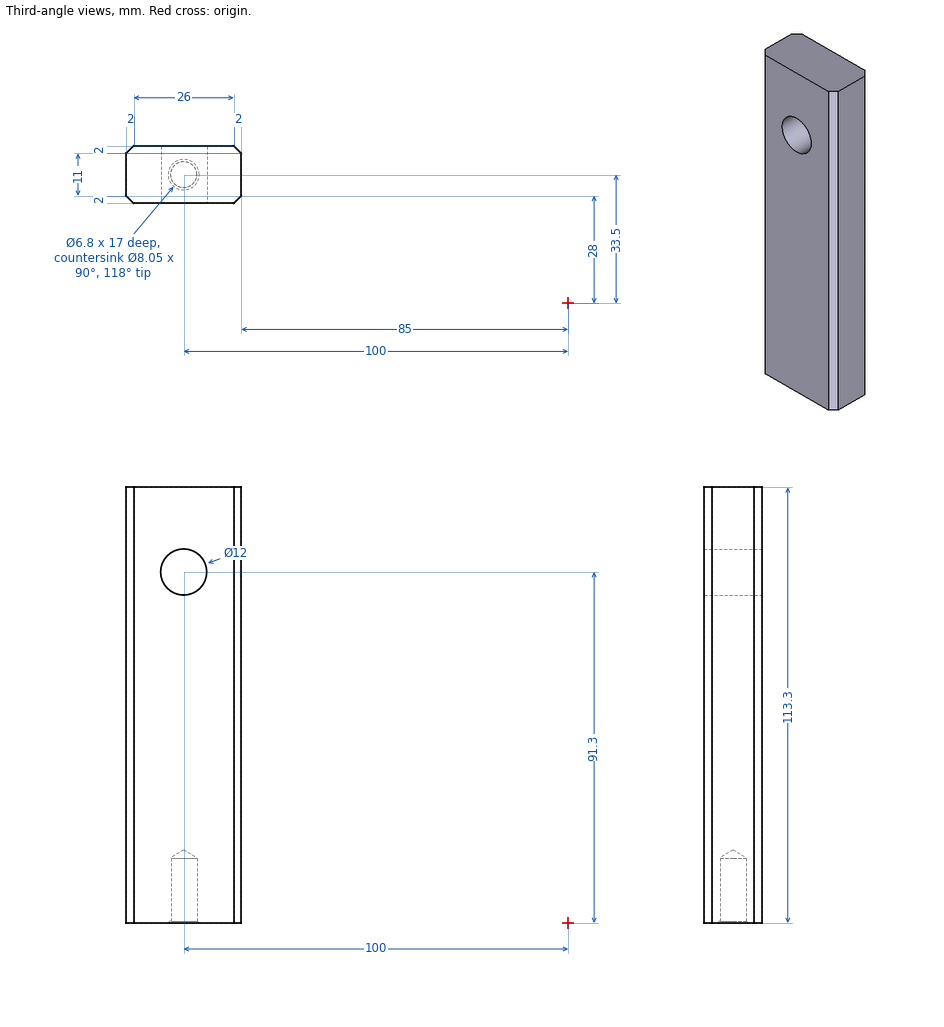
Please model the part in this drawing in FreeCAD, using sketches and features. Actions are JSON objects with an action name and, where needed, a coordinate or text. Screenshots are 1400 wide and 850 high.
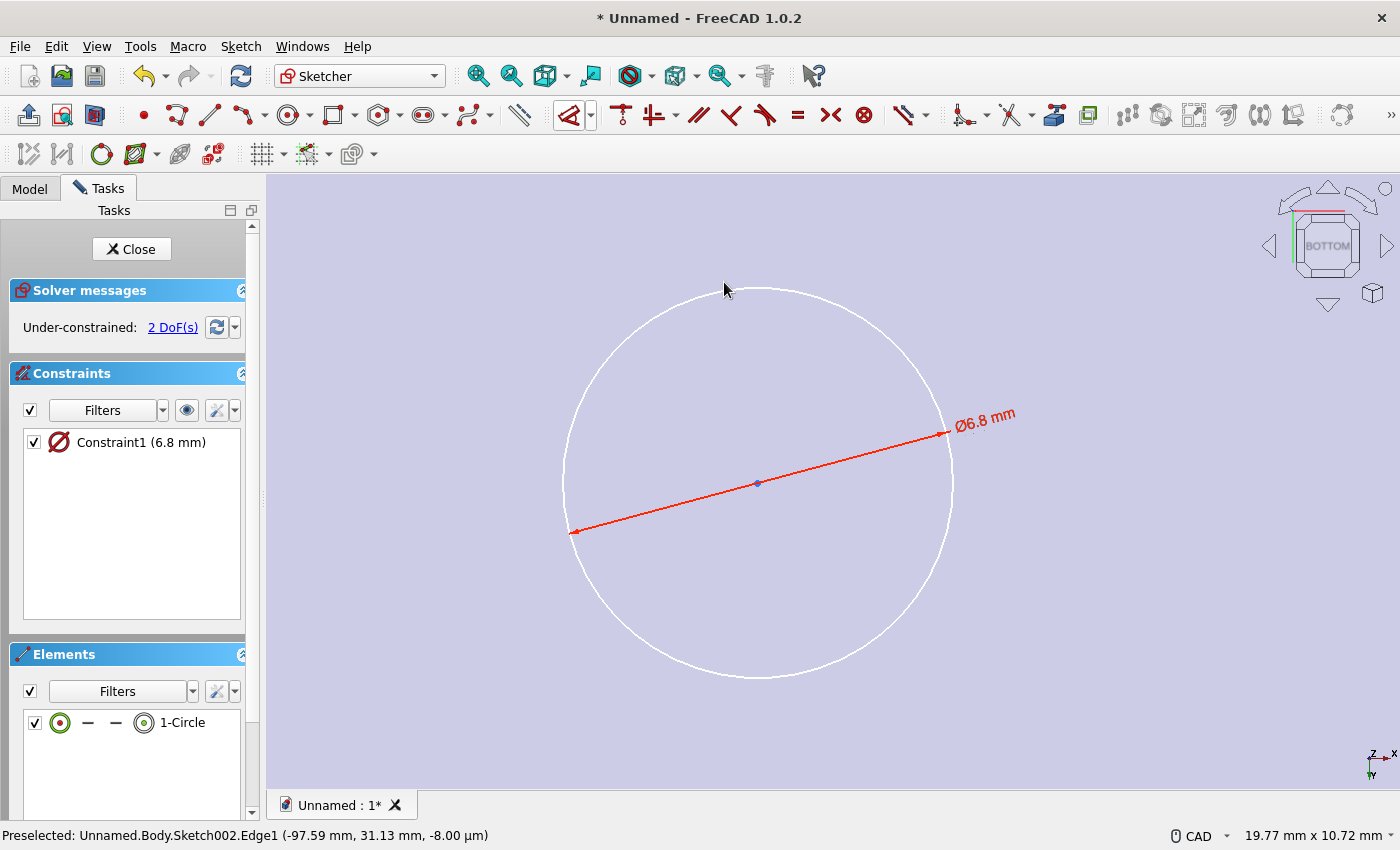
{"action": "left_click", "coordinate": [758, 483]}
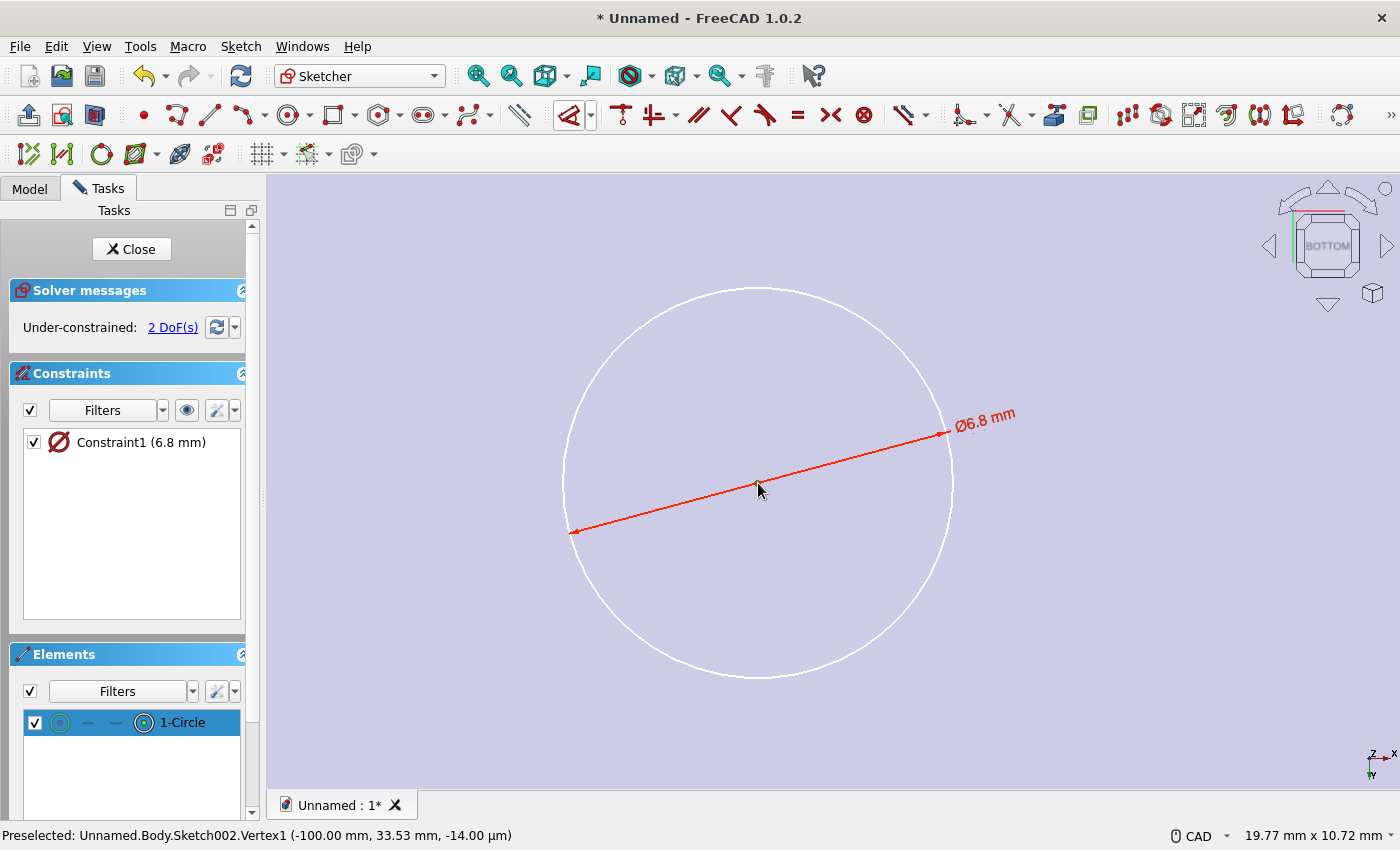
{"action": "left_click", "coordinate": [590, 116]}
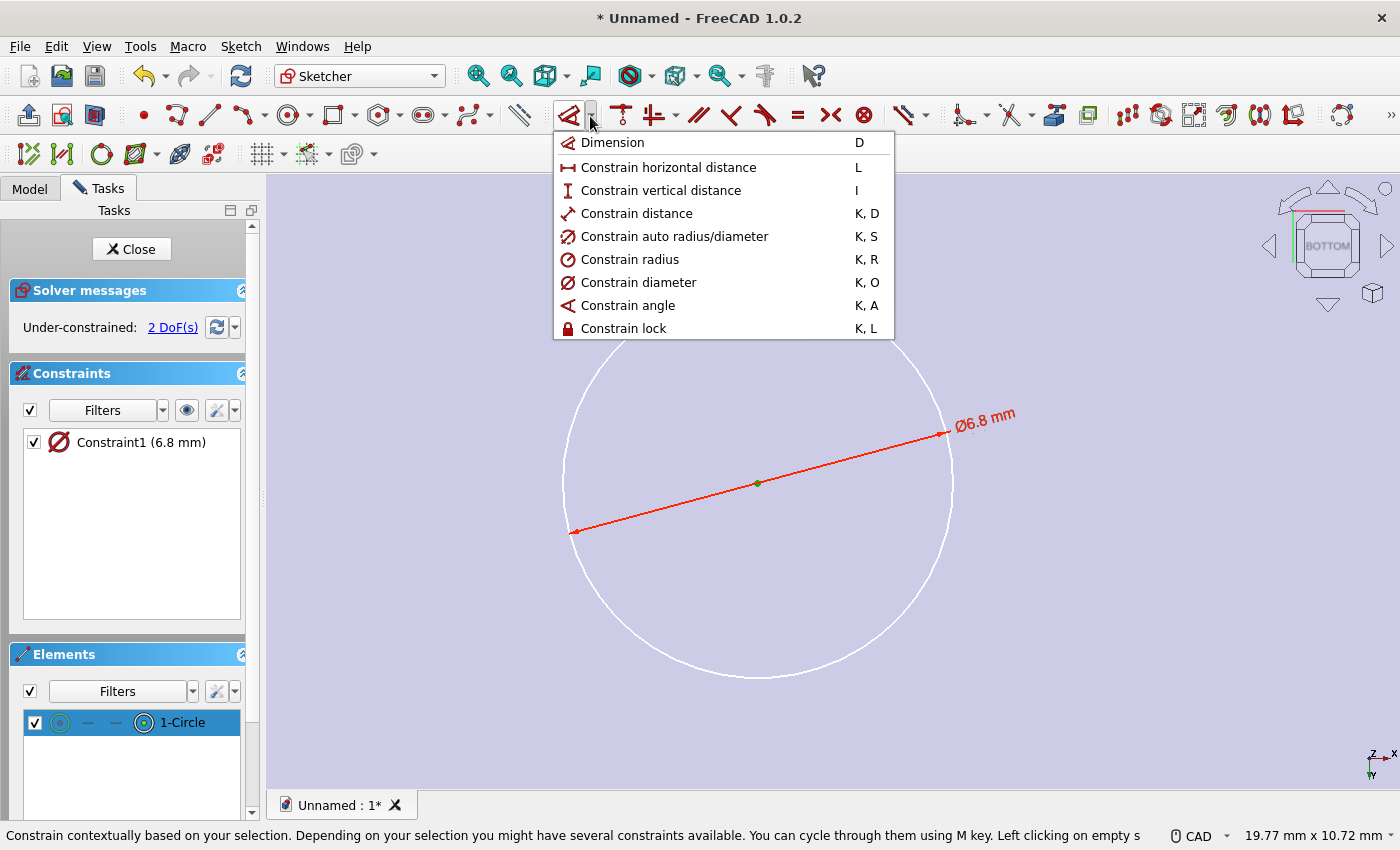
{"action": "left_click", "coordinate": [724, 168]}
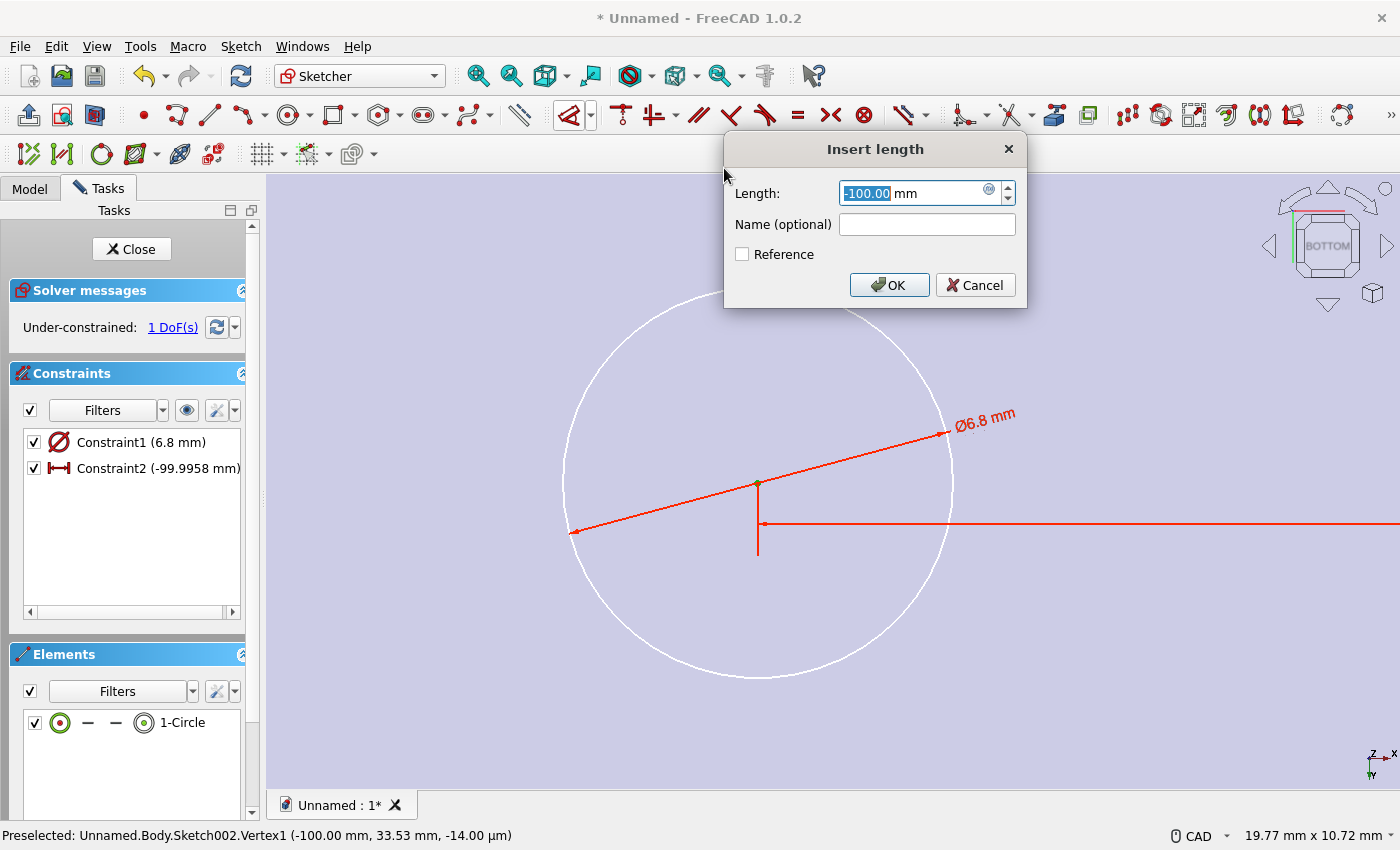
{"action": "type", "text": "-100"}
{"action": "key", "text": "Return"}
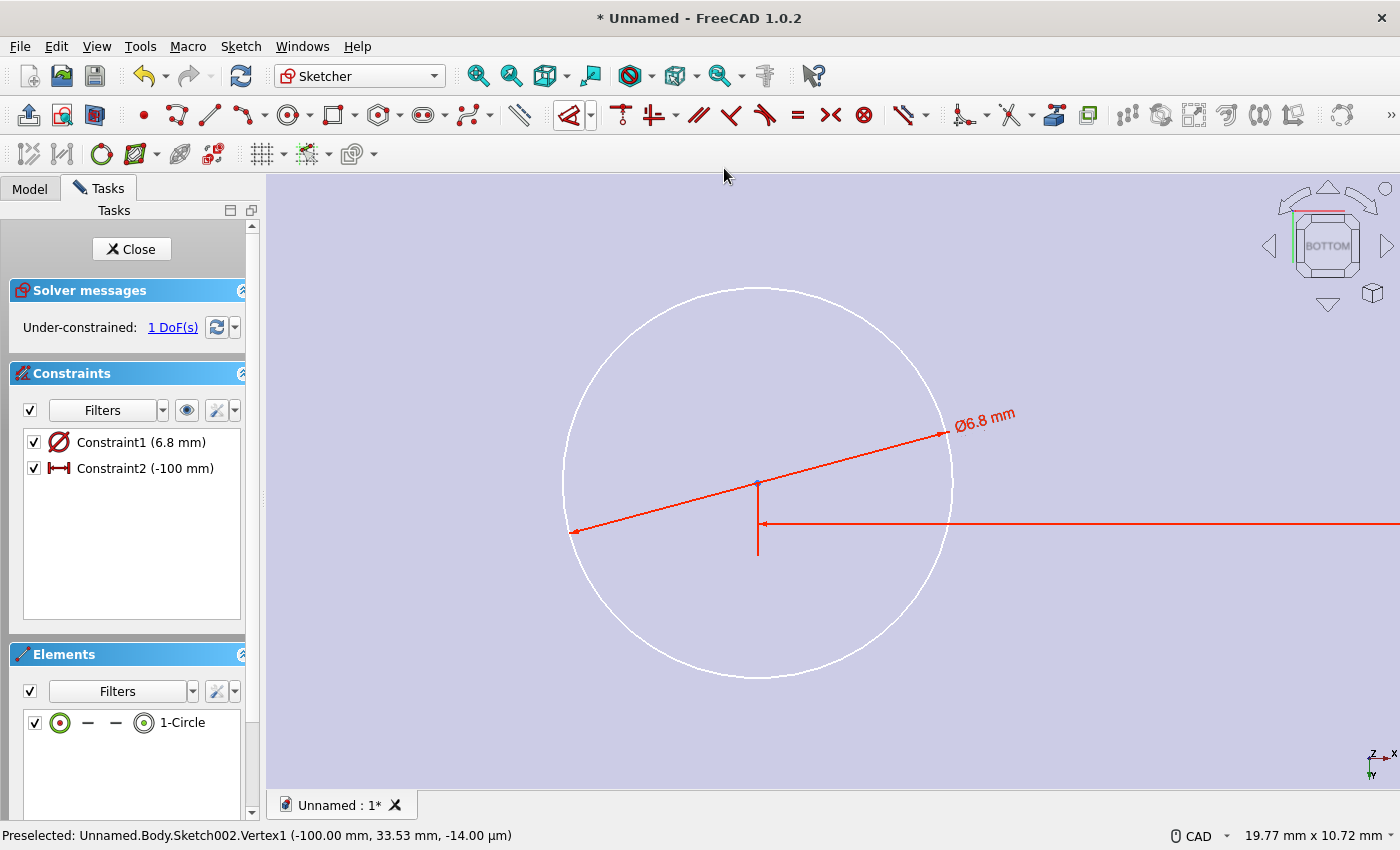
{"action": "left_click", "coordinate": [758, 483]}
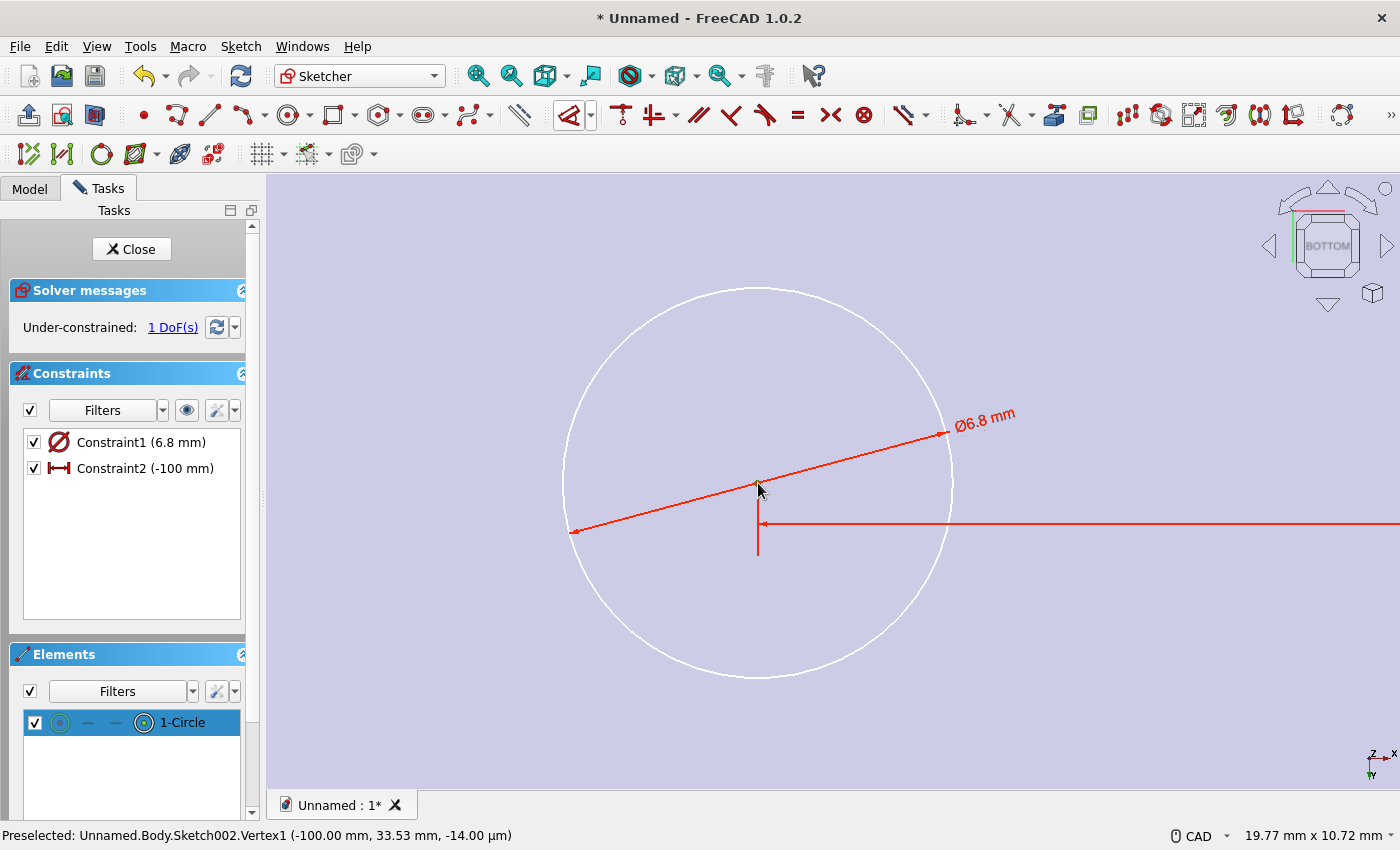
{"action": "left_click", "coordinate": [590, 116]}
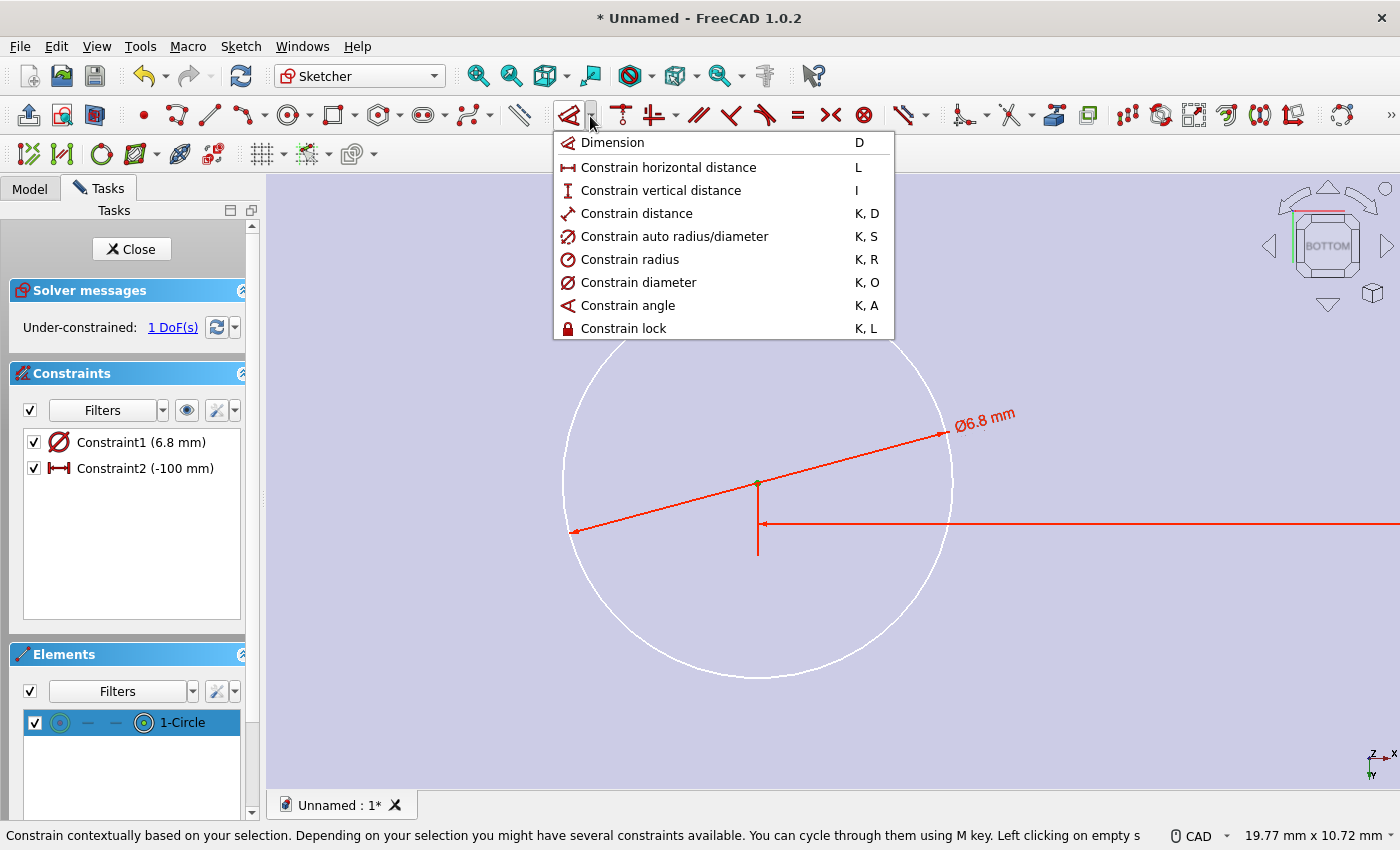
{"action": "left_click", "coordinate": [724, 190]}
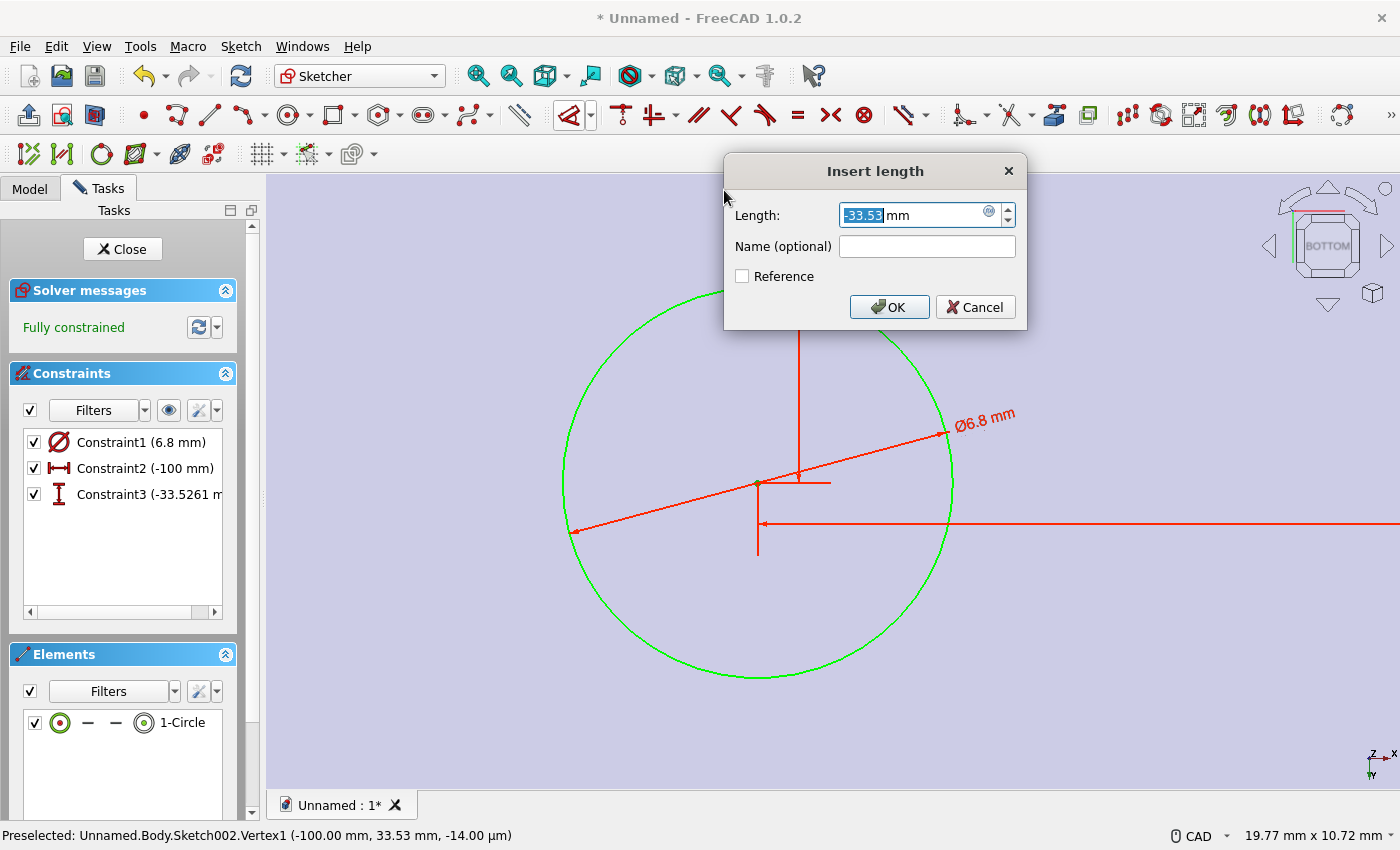
{"action": "type", "text": "-33.5"}
{"action": "key", "text": "Return"}